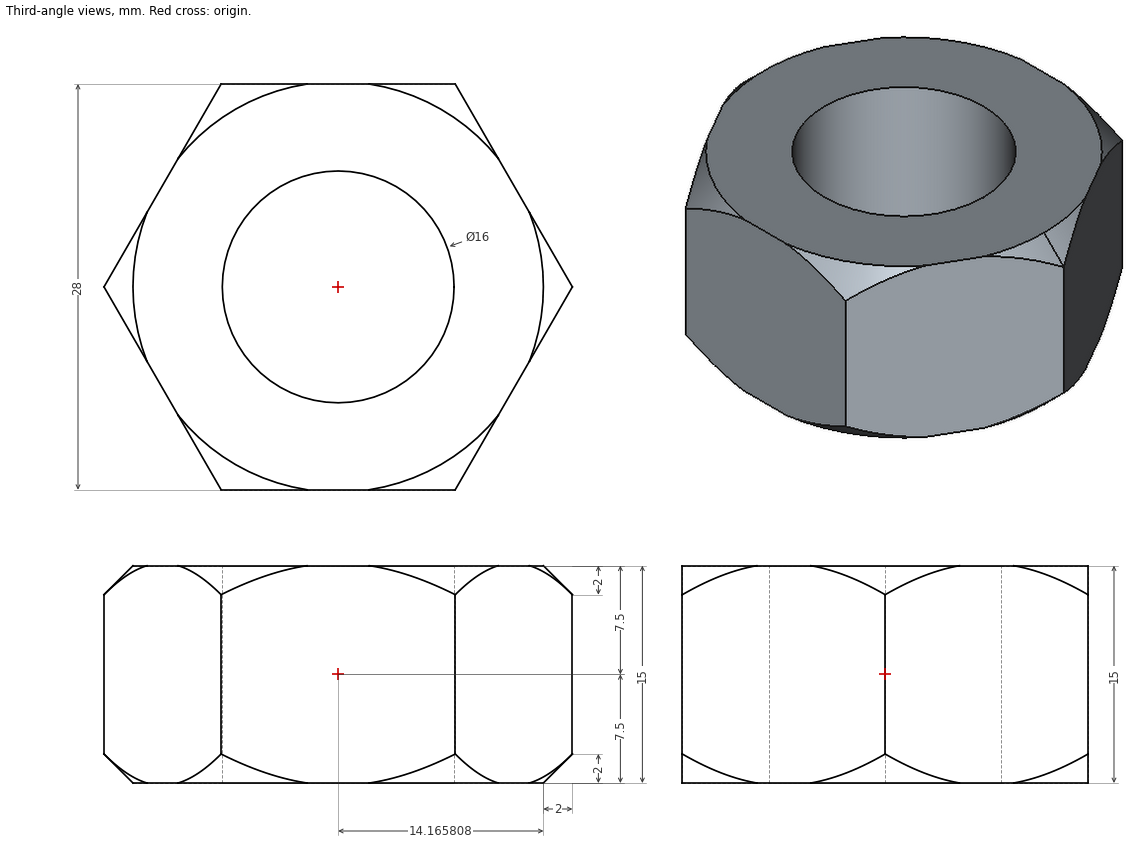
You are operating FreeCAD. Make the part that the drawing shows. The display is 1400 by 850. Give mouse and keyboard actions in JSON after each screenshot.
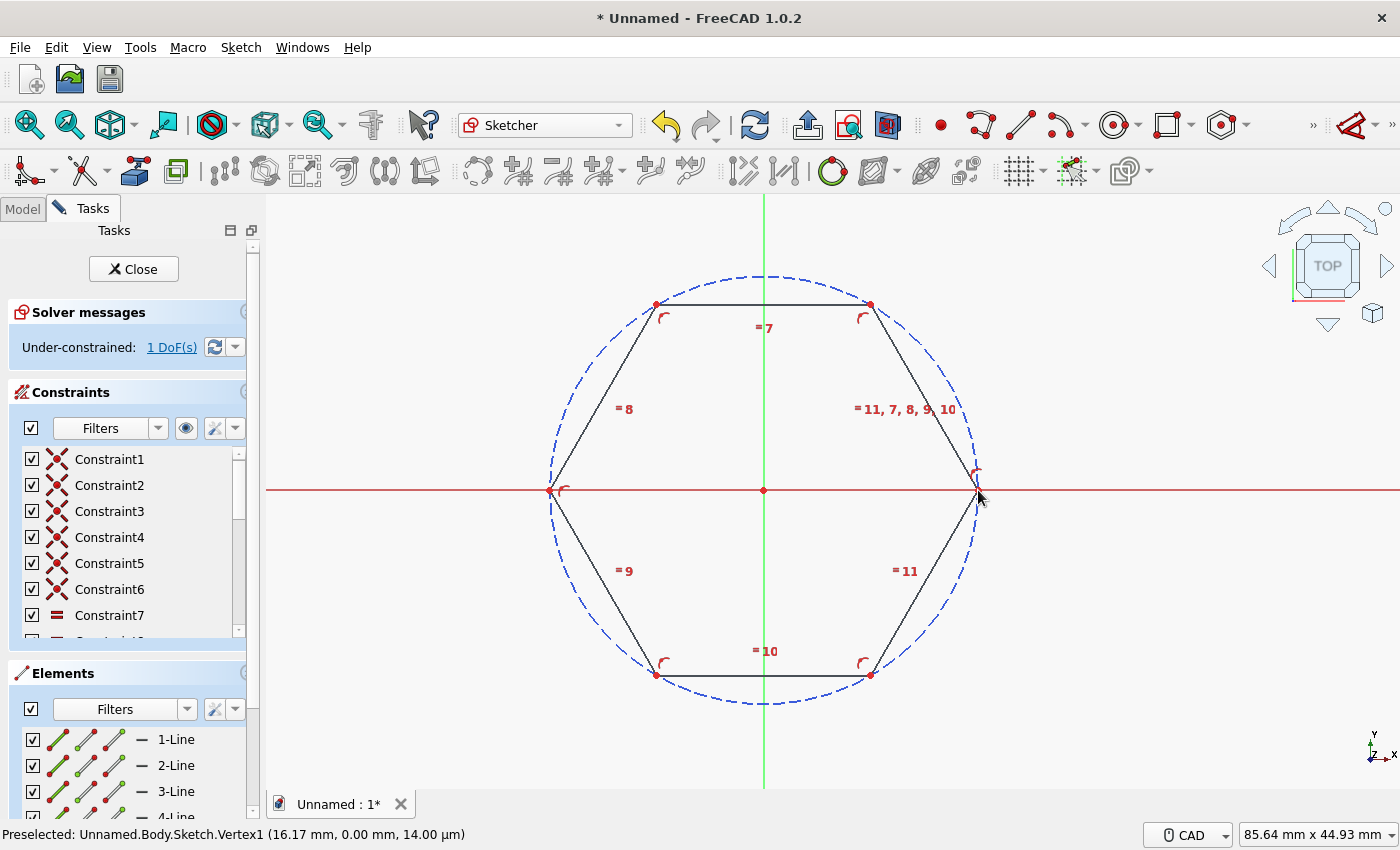
{"action": "left_click", "coordinate": [1352, 126]}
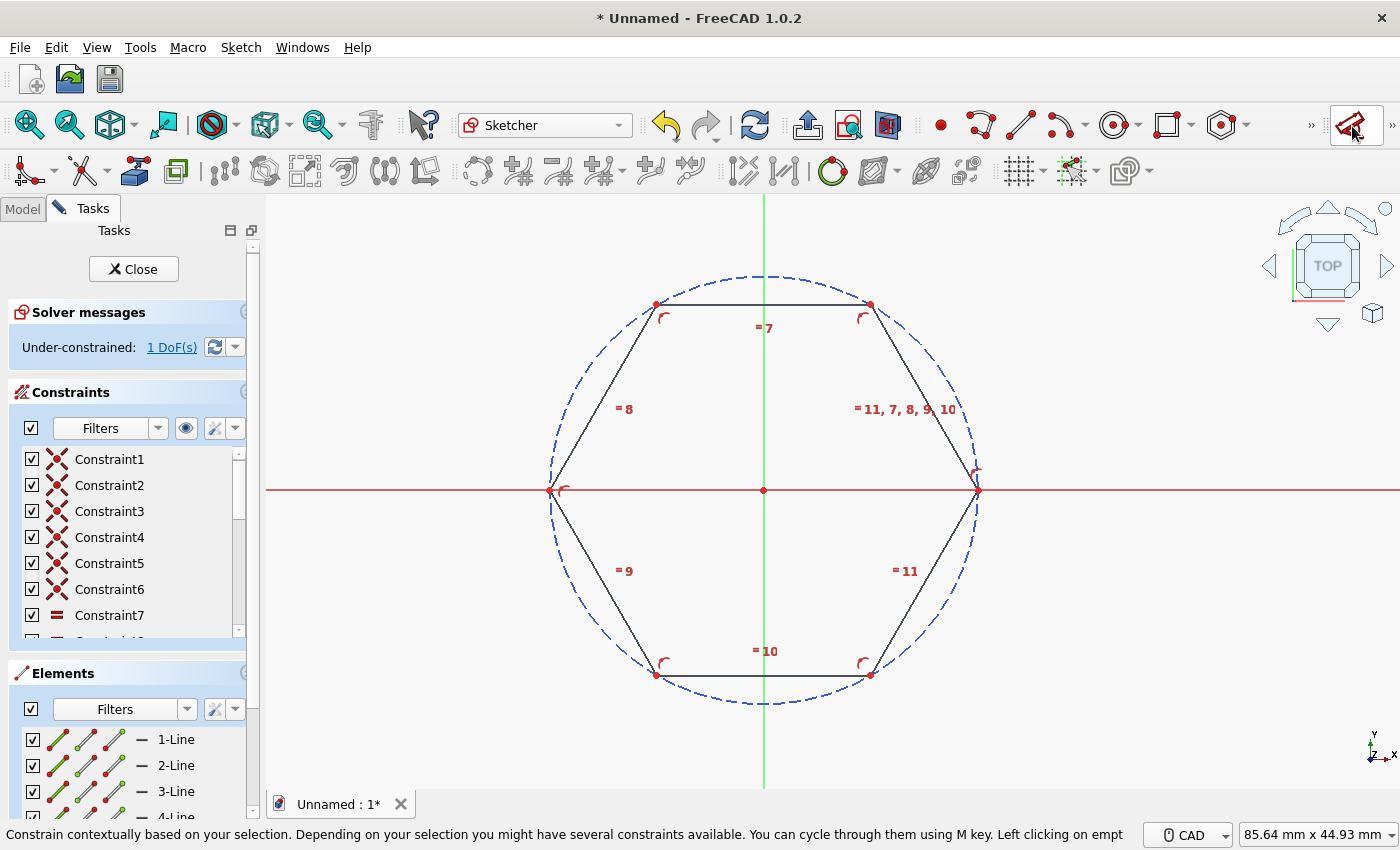
{"action": "left_click", "coordinate": [657, 676]}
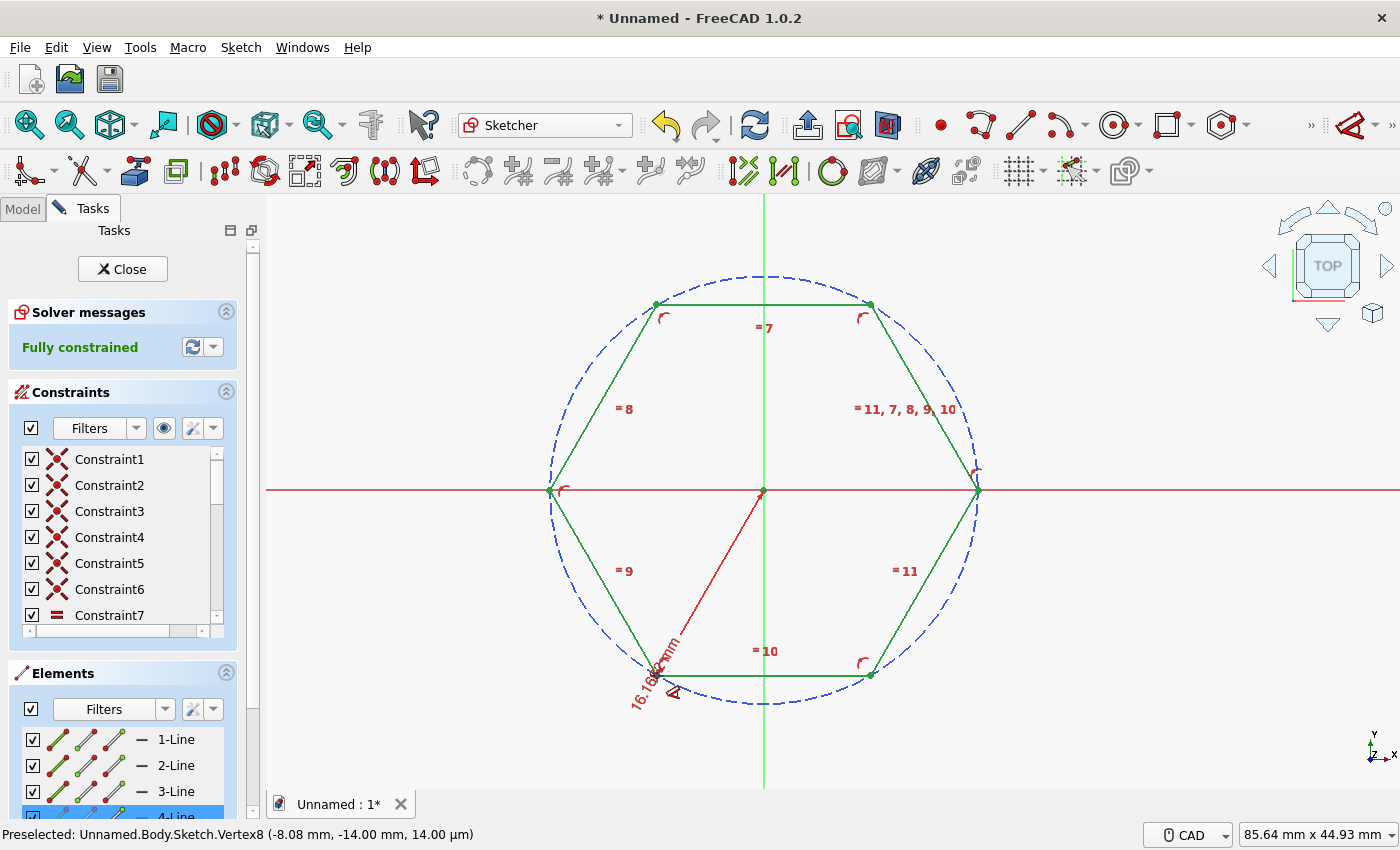
{"action": "left_click", "coordinate": [871, 305]}
{"action": "left_click", "coordinate": [905, 405]}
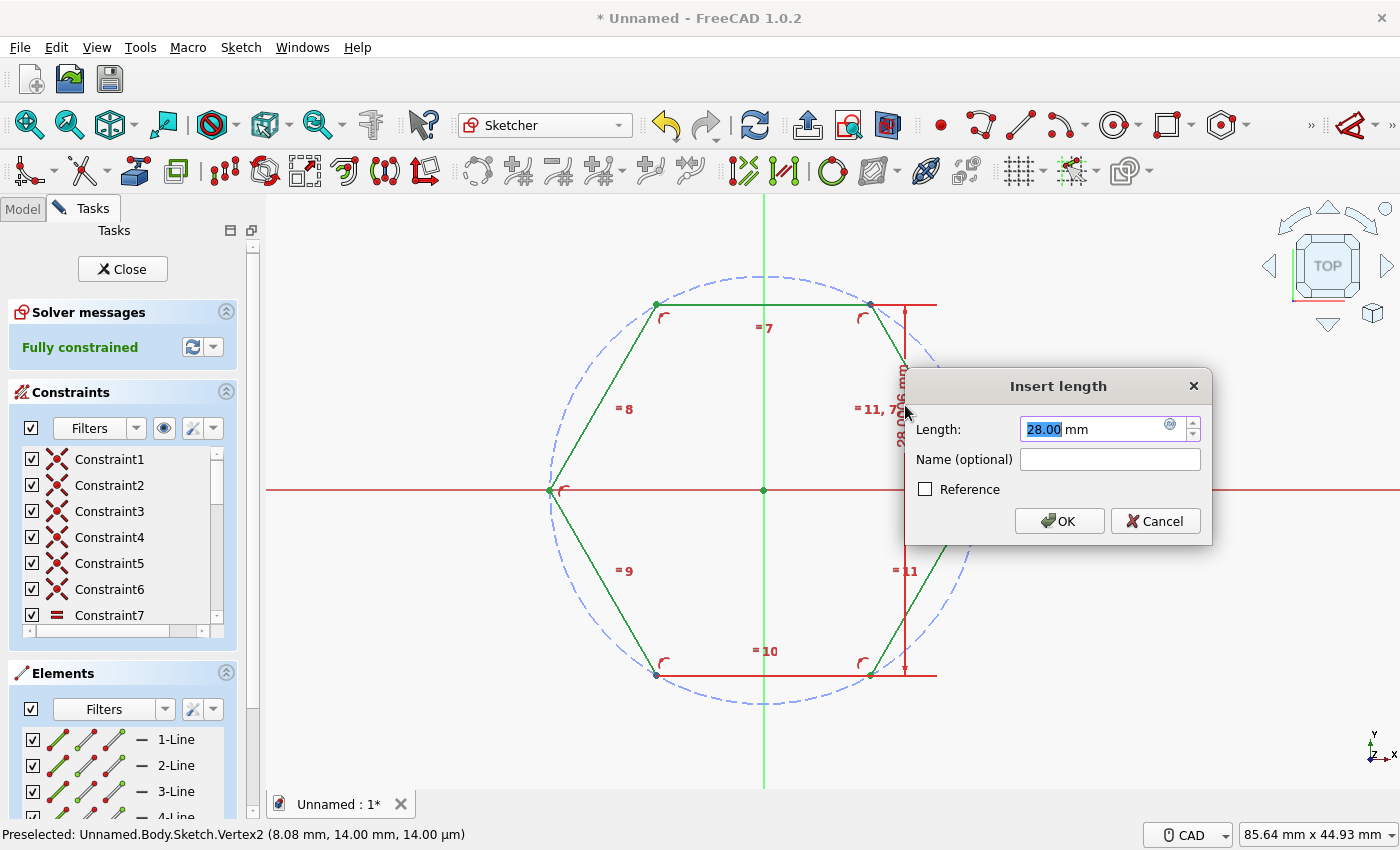
{"action": "type", "text": "28"}
{"action": "key", "text": "Return"}
{"action": "key", "text": "Escape"}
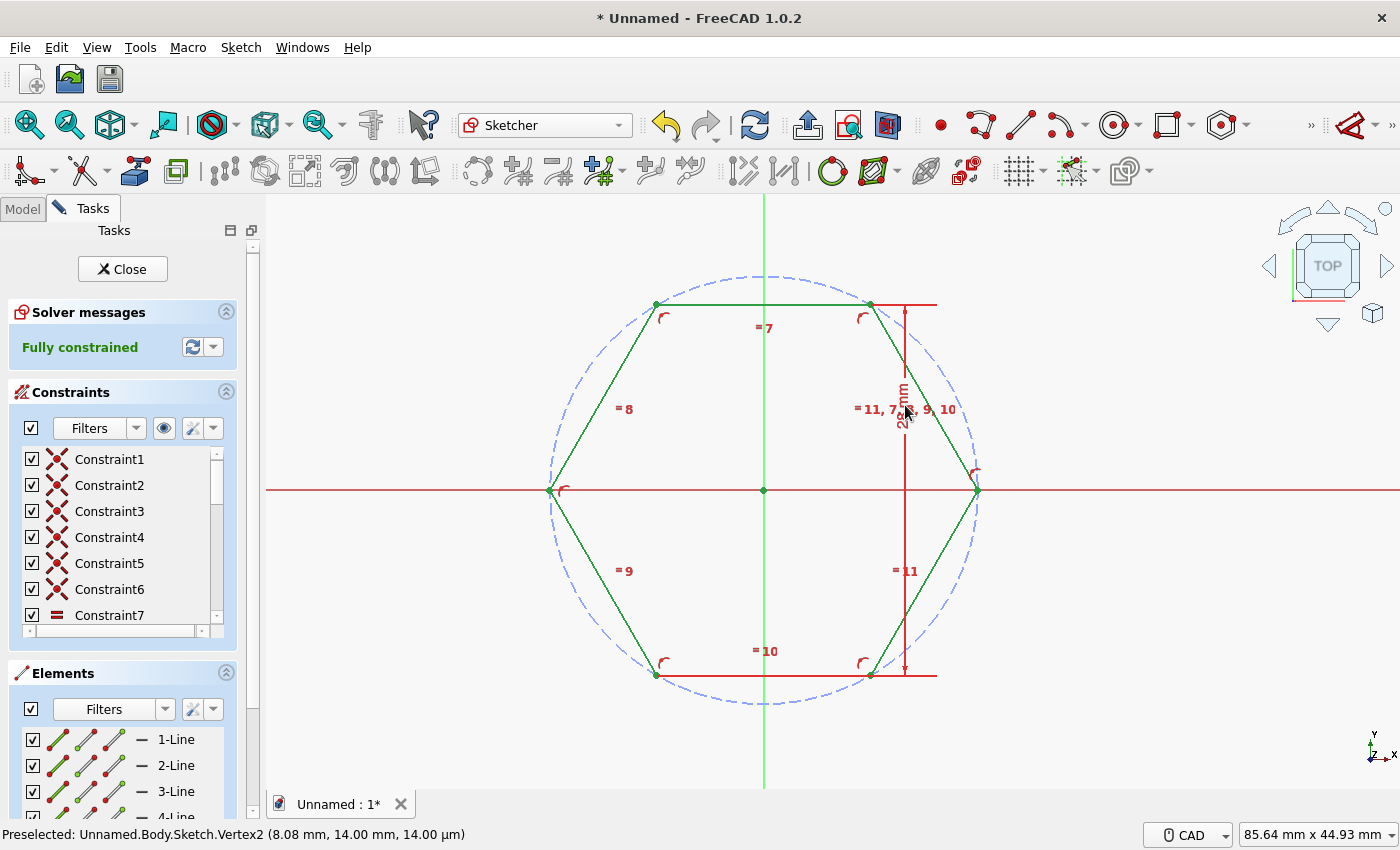
{"action": "left_click", "coordinate": [123, 269]}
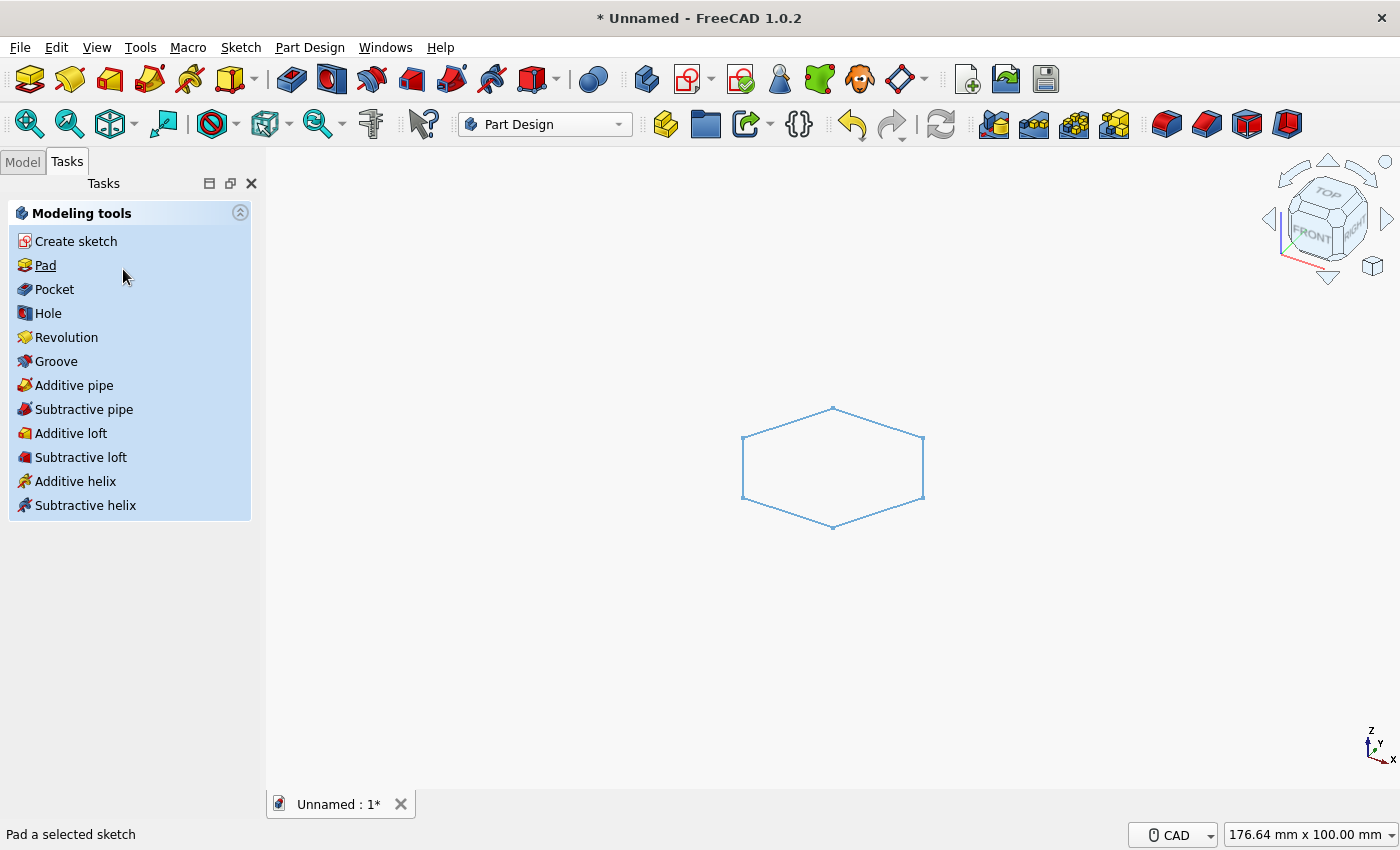
{"action": "left_click", "coordinate": [30, 80]}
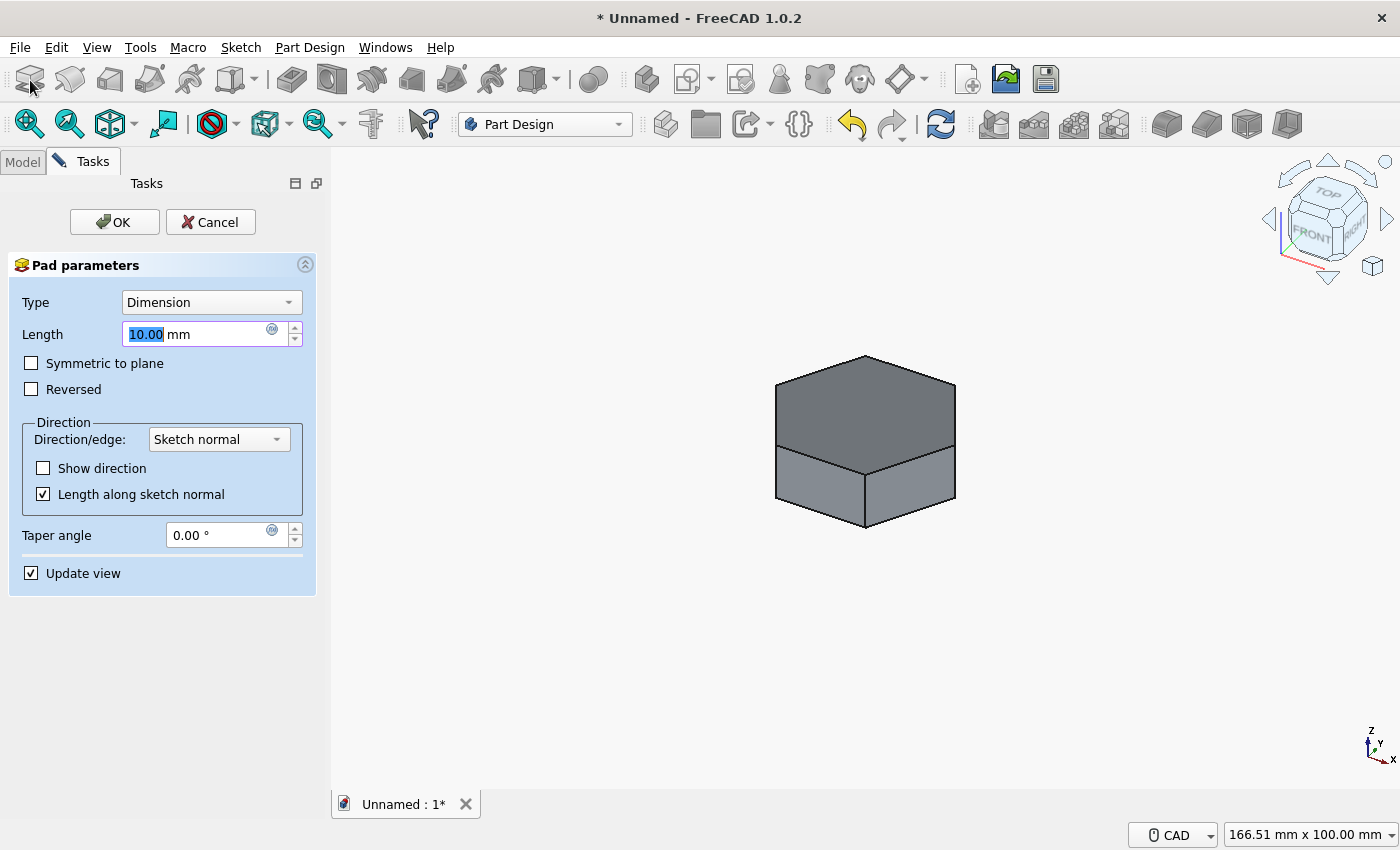
{"action": "type", "text": "15"}
{"action": "key", "text": "Tab"}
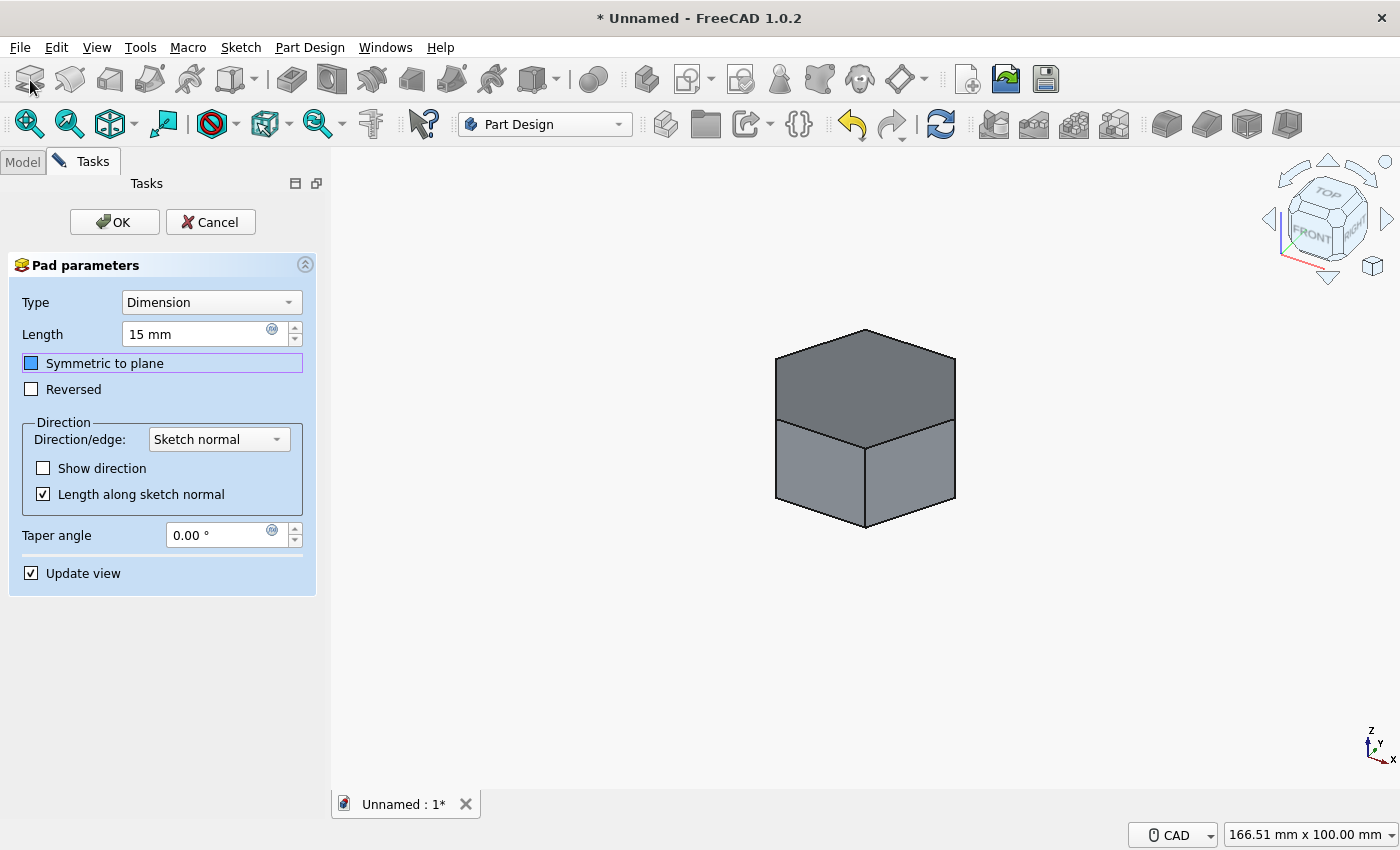
{"action": "left_click", "coordinate": [30, 363]}